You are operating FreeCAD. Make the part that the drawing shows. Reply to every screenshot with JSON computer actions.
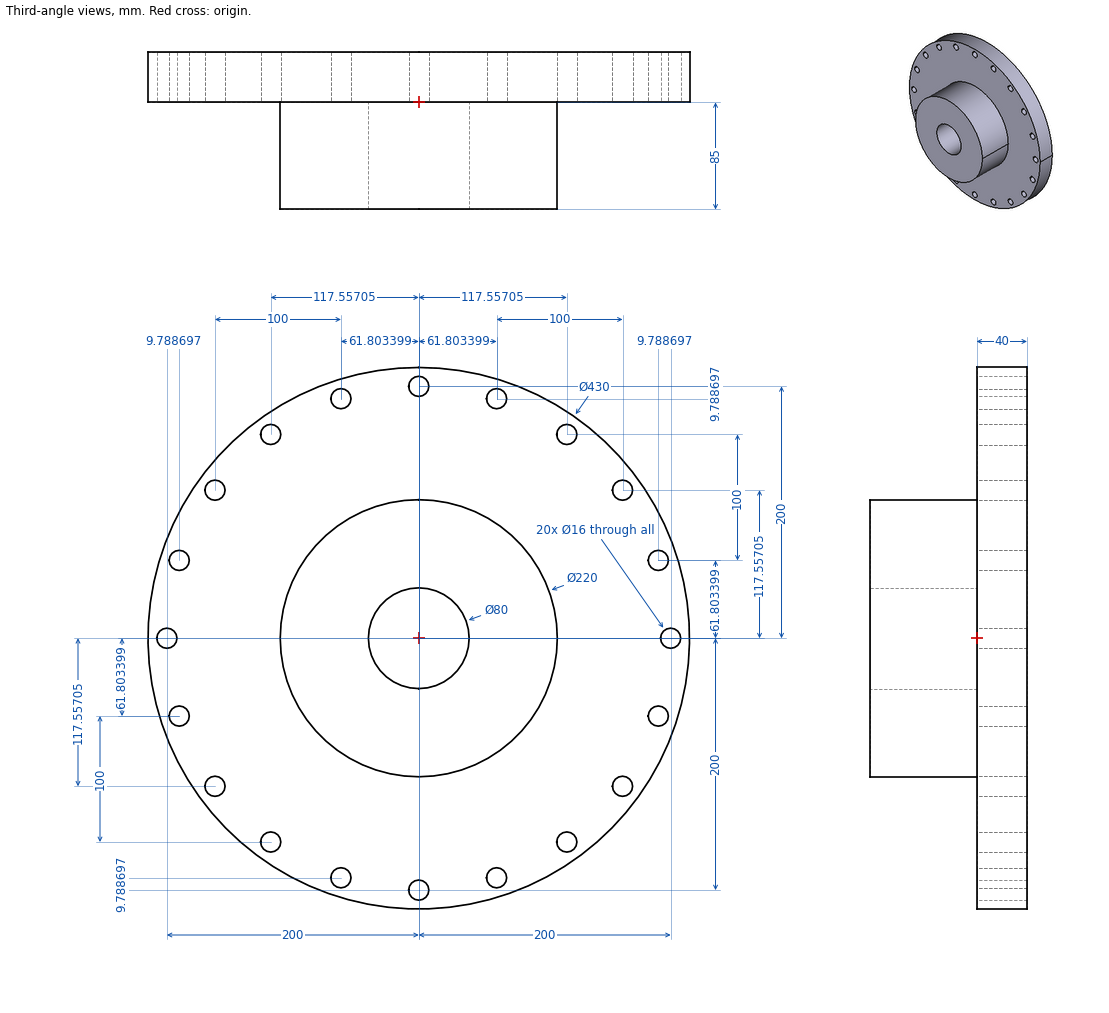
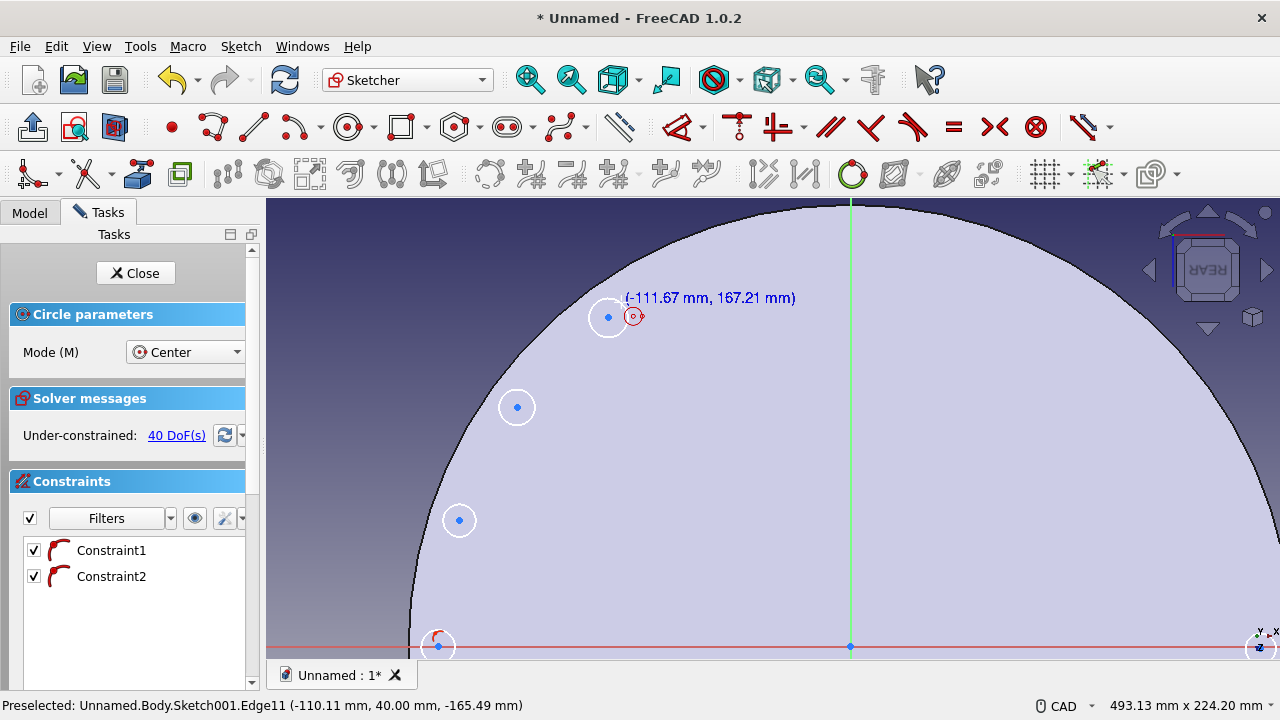
{"action": "scroll", "coordinate": [724, 256], "scroll_direction": "up", "scroll_amount": 2}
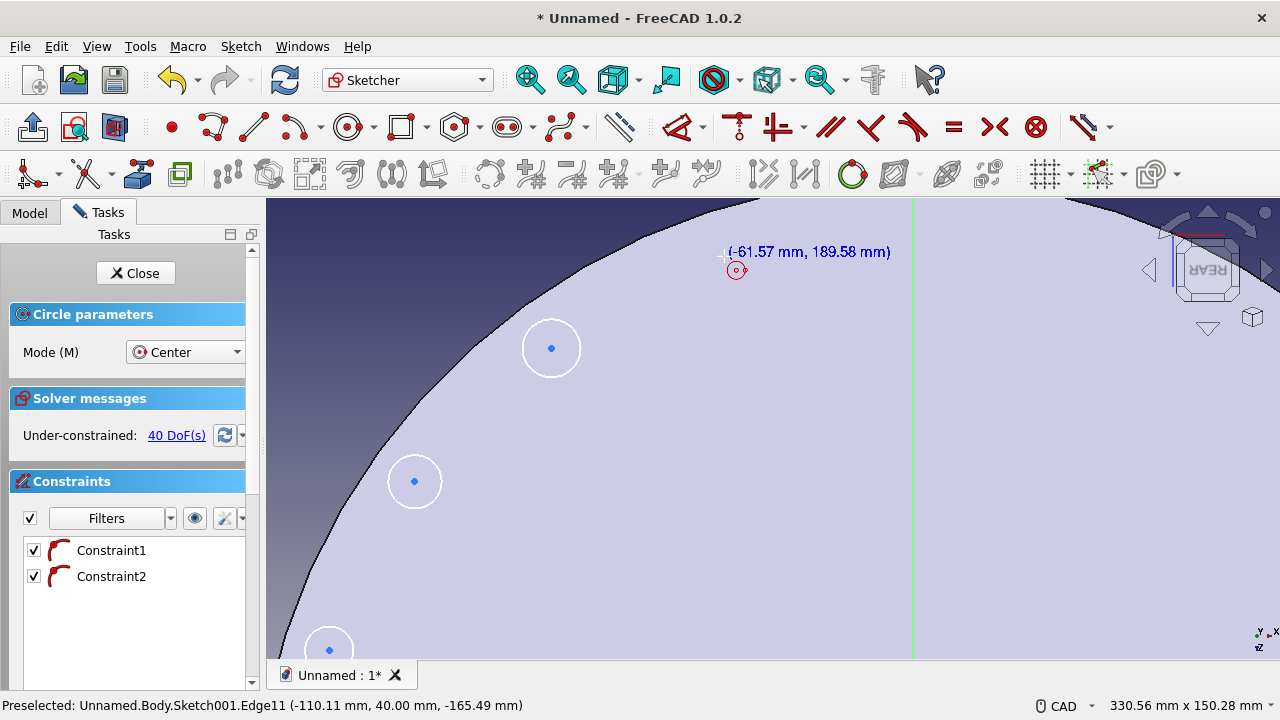
{"action": "scroll", "coordinate": [636, 294], "scroll_direction": "down", "scroll_amount": 7}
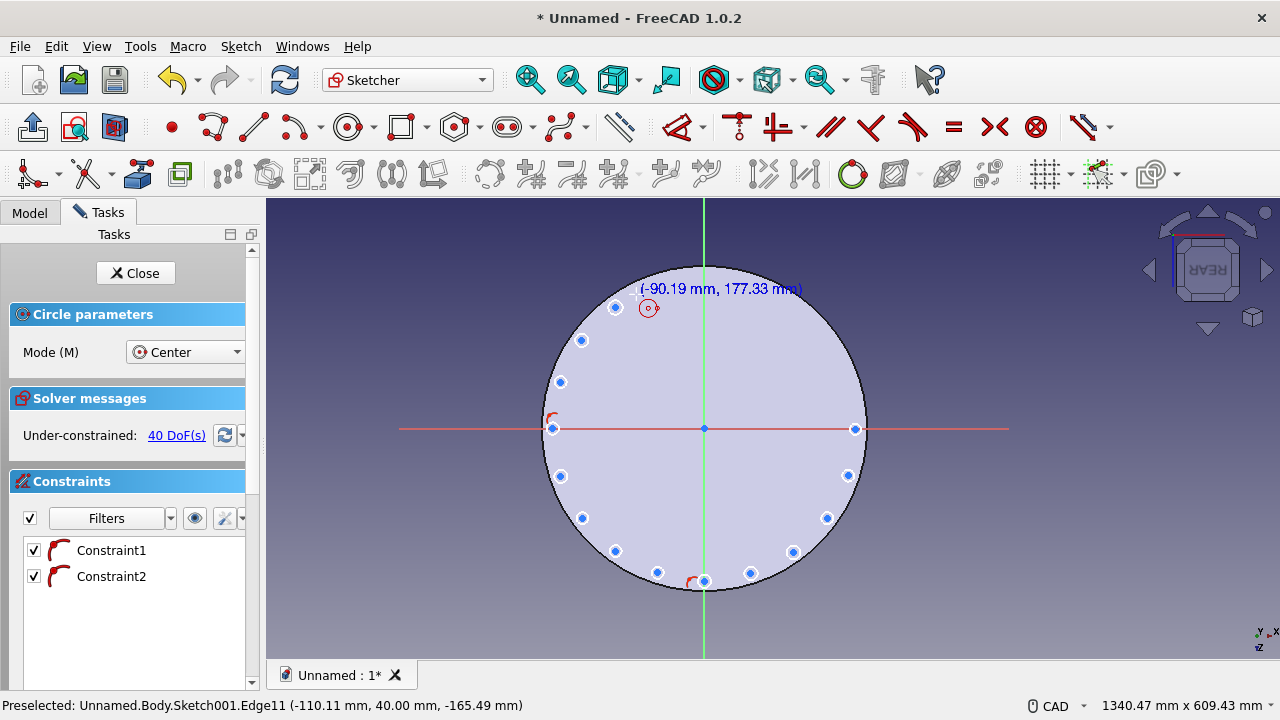
{"action": "left_click", "coordinate": [658, 285]}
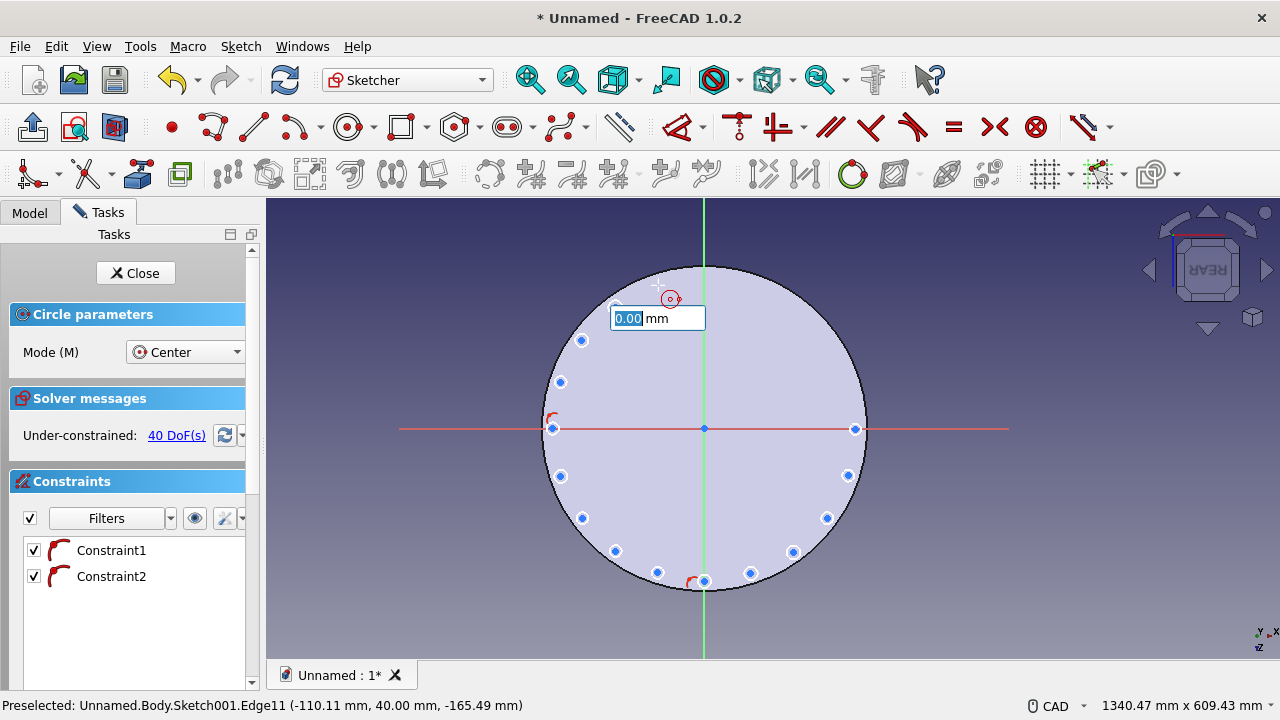
{"action": "scroll", "coordinate": [662, 280], "scroll_direction": "up", "scroll_amount": 5}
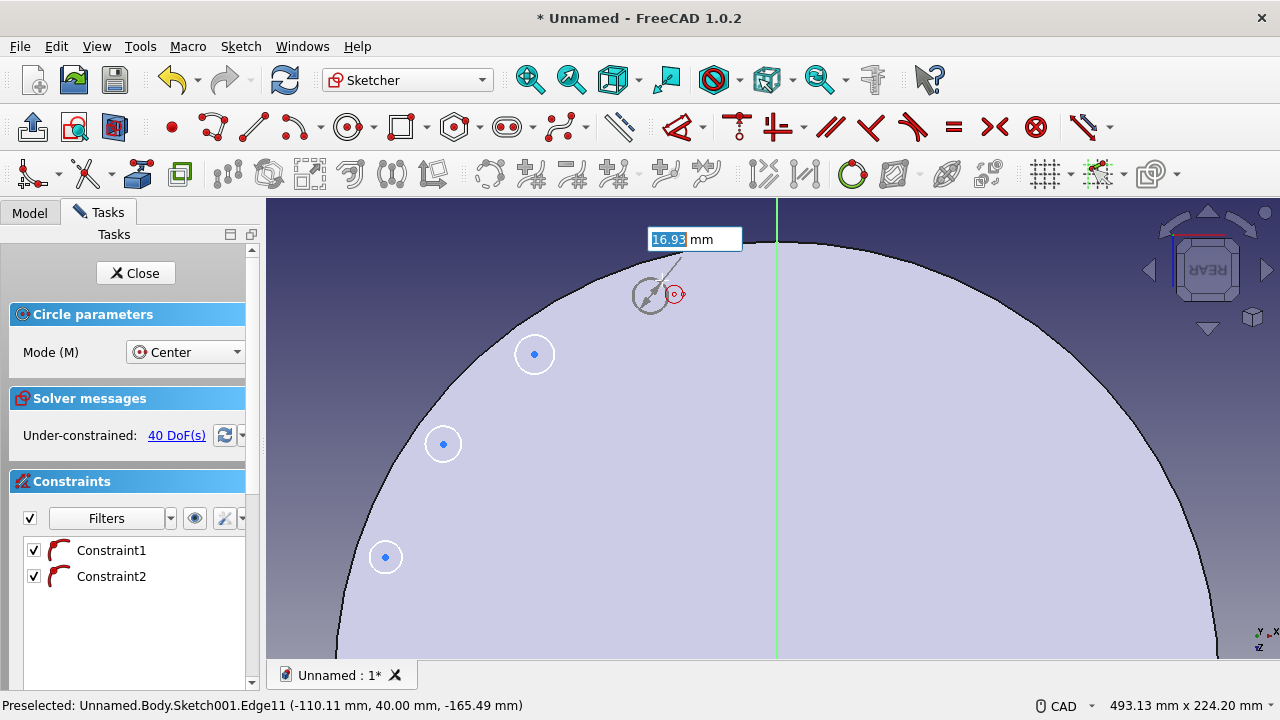
{"action": "left_click", "coordinate": [661, 281]}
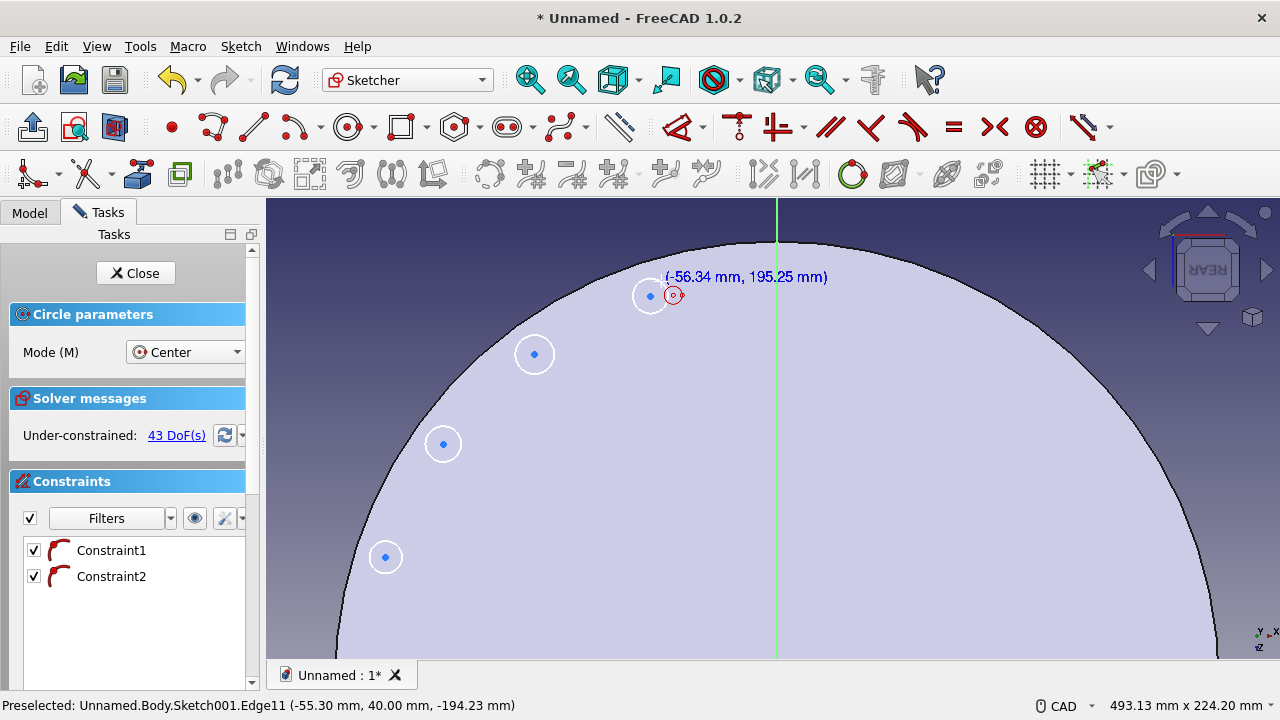
{"action": "scroll", "coordinate": [777, 272], "scroll_direction": "up", "scroll_amount": 2}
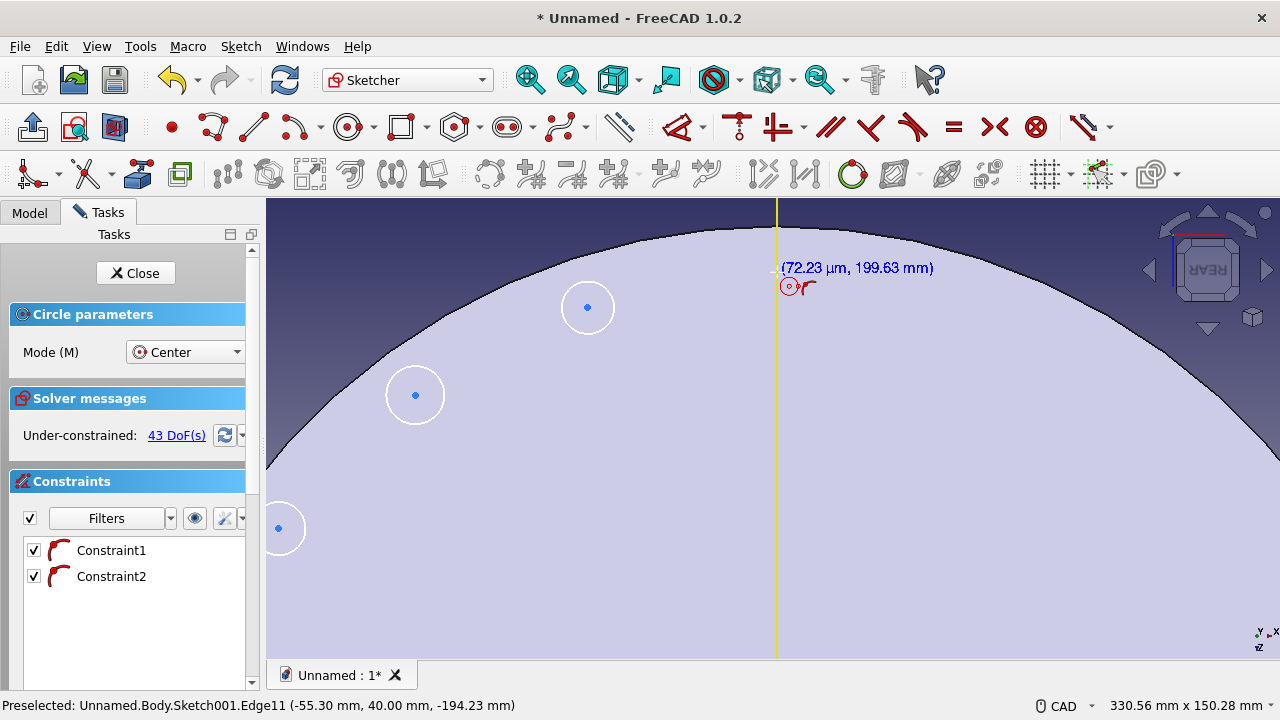
{"action": "scroll", "coordinate": [681, 279], "scroll_direction": "down", "scroll_amount": 7}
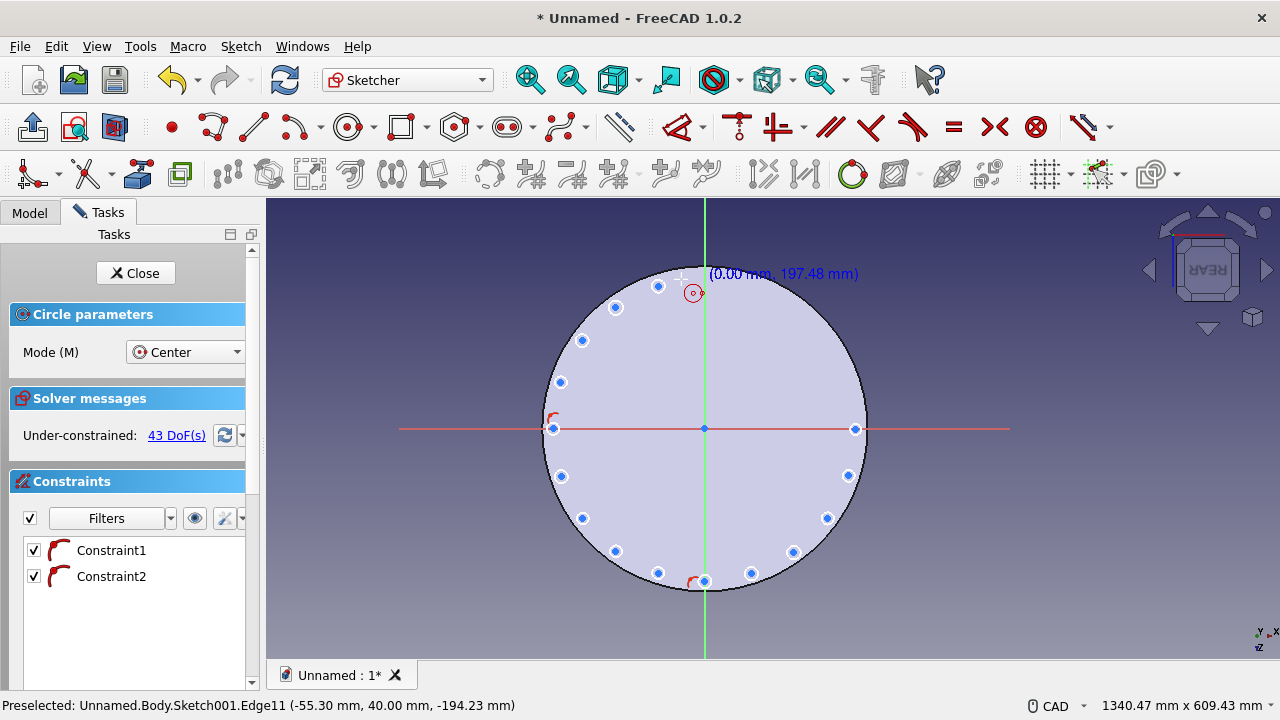
{"action": "left_click", "coordinate": [705, 277]}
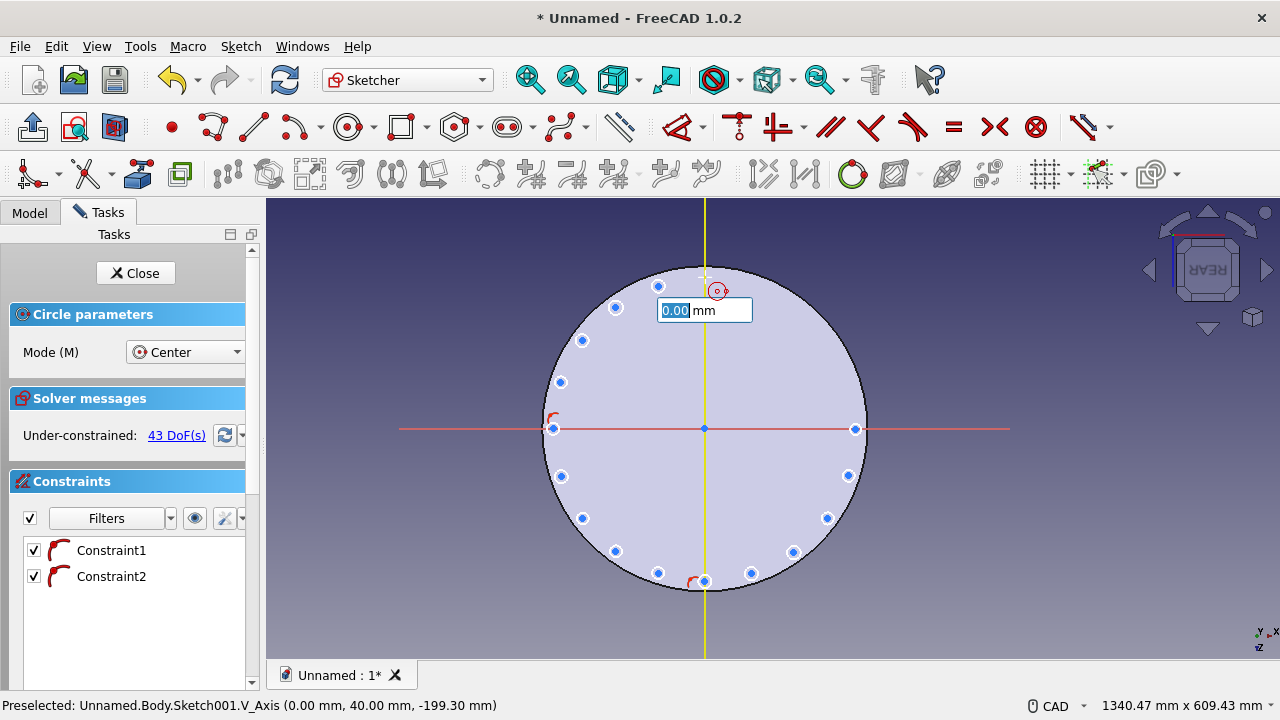
{"action": "scroll", "coordinate": [711, 275], "scroll_direction": "up", "scroll_amount": 6}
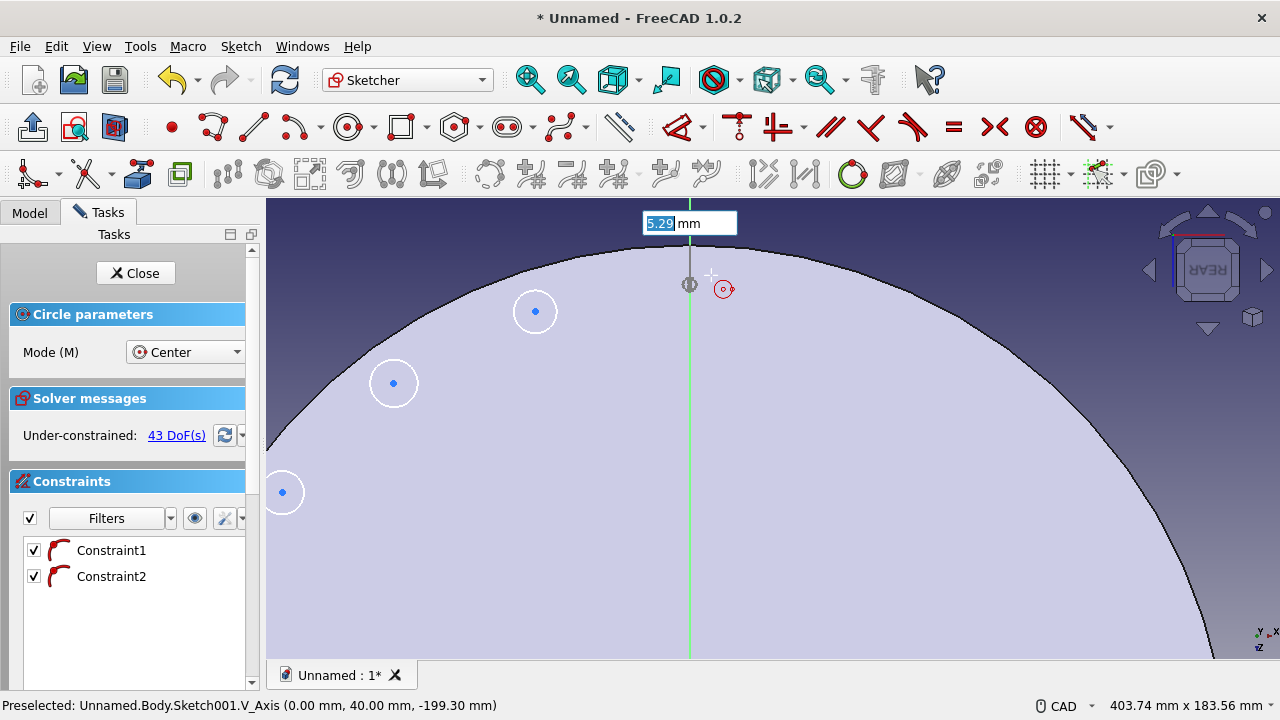
{"action": "left_click", "coordinate": [708, 276]}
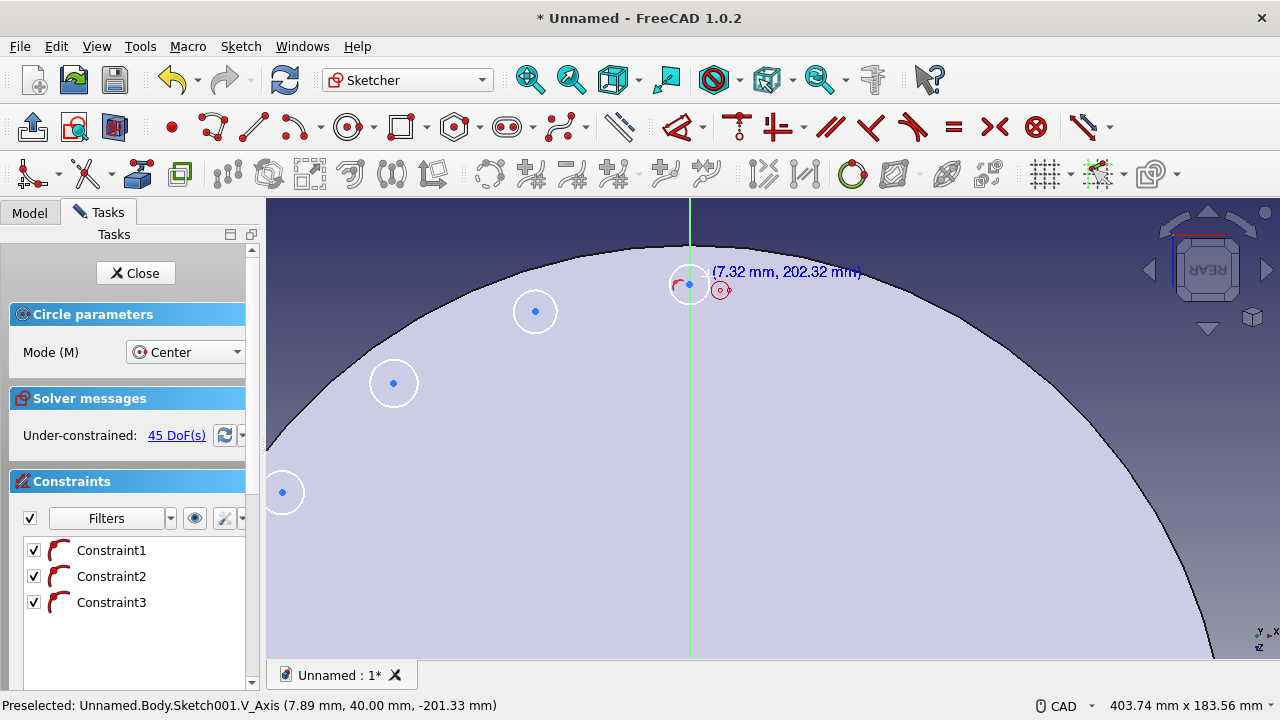
{"action": "left_click", "coordinate": [845, 307]}
{"action": "left_click", "coordinate": [859, 293]}